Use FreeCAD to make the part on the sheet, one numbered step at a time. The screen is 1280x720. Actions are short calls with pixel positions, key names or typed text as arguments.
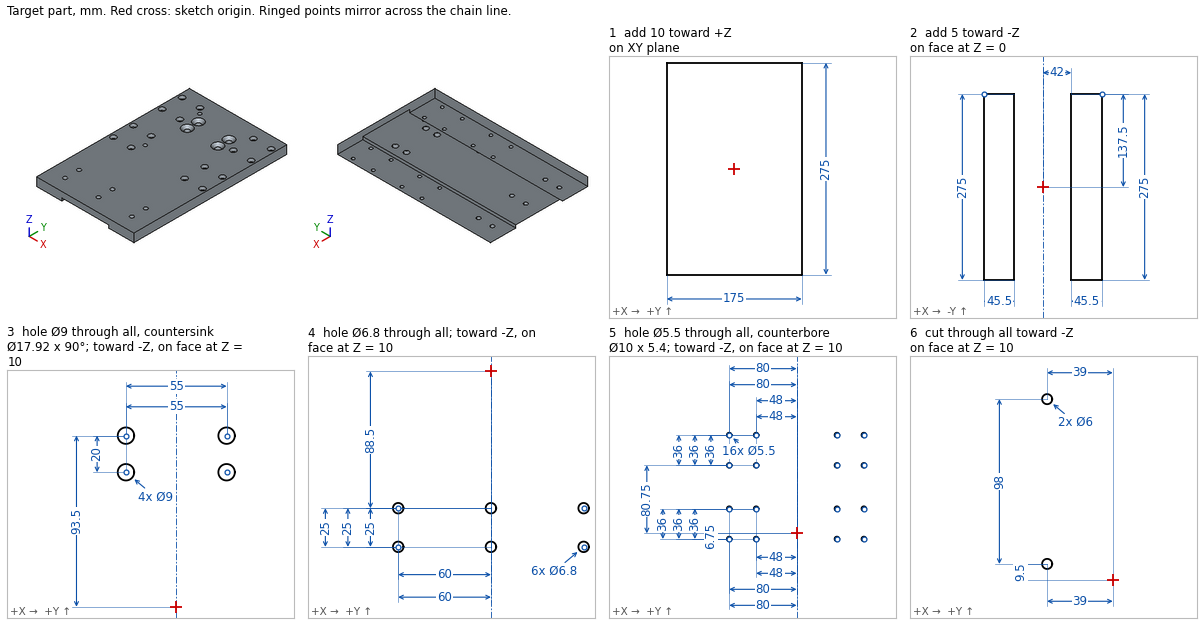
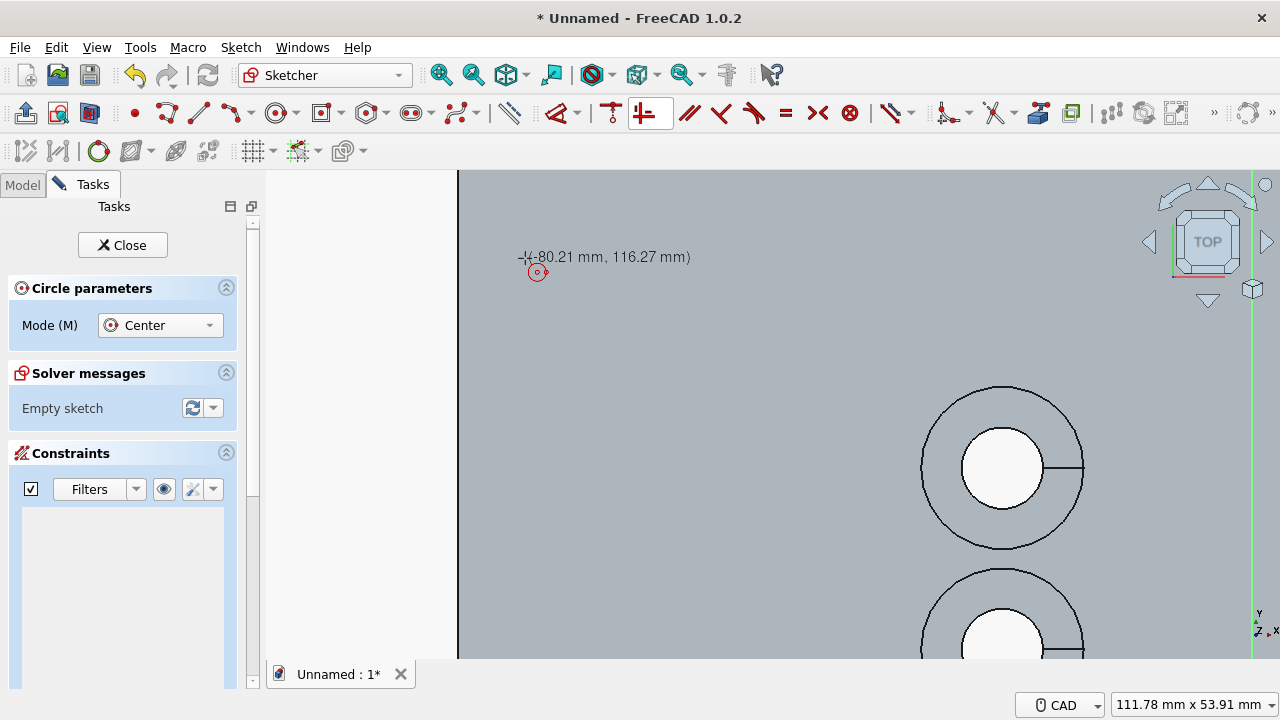
scroll(525, 283, down, 7)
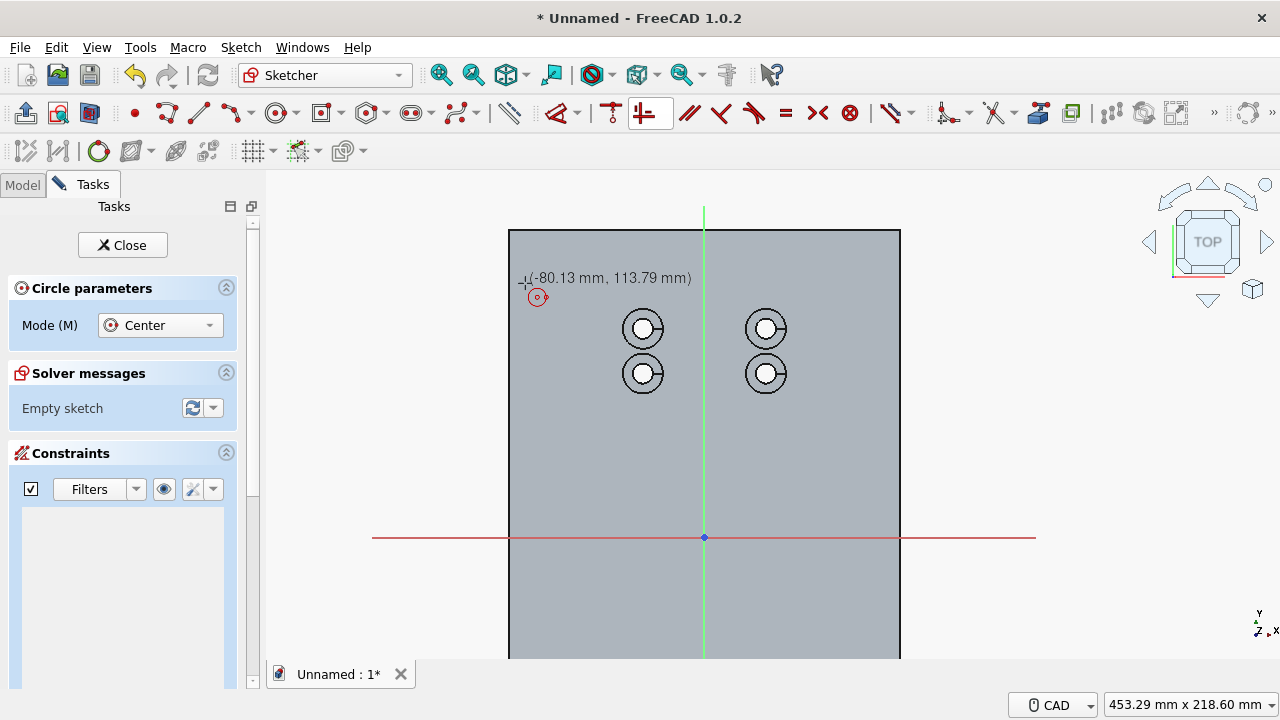
click(525, 277)
move(530, 272)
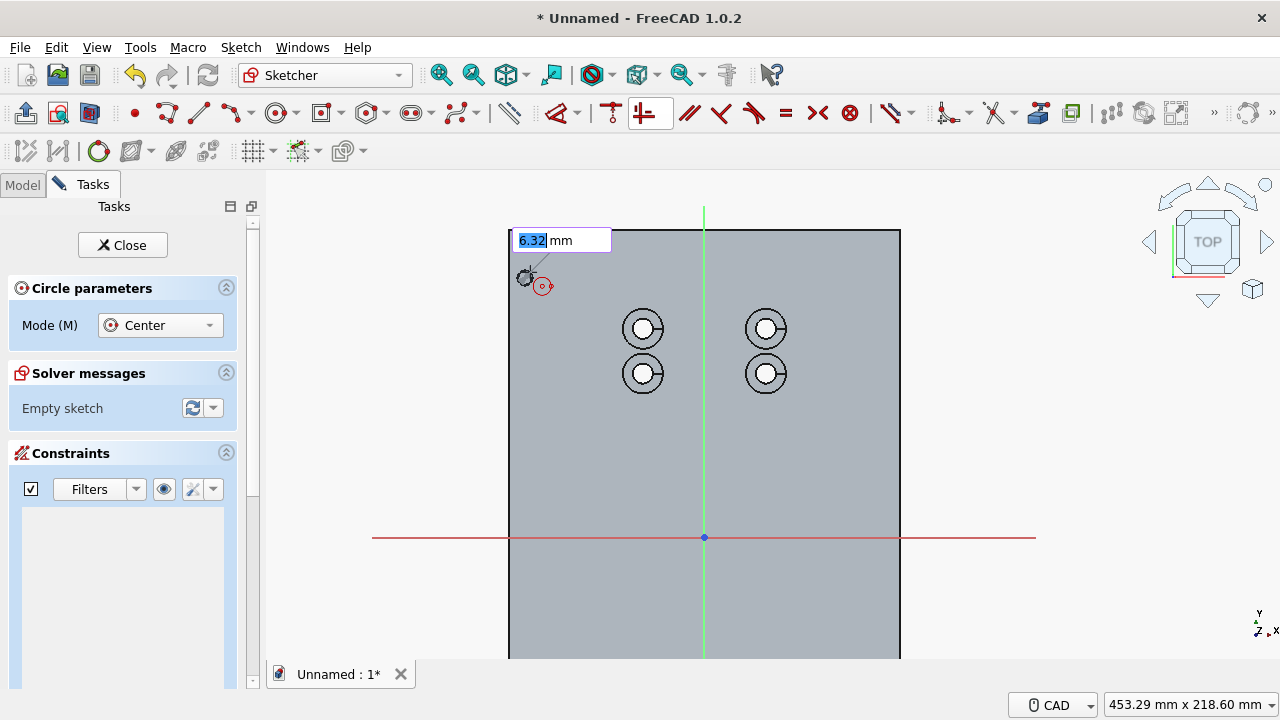
text(5.5)
key(Return)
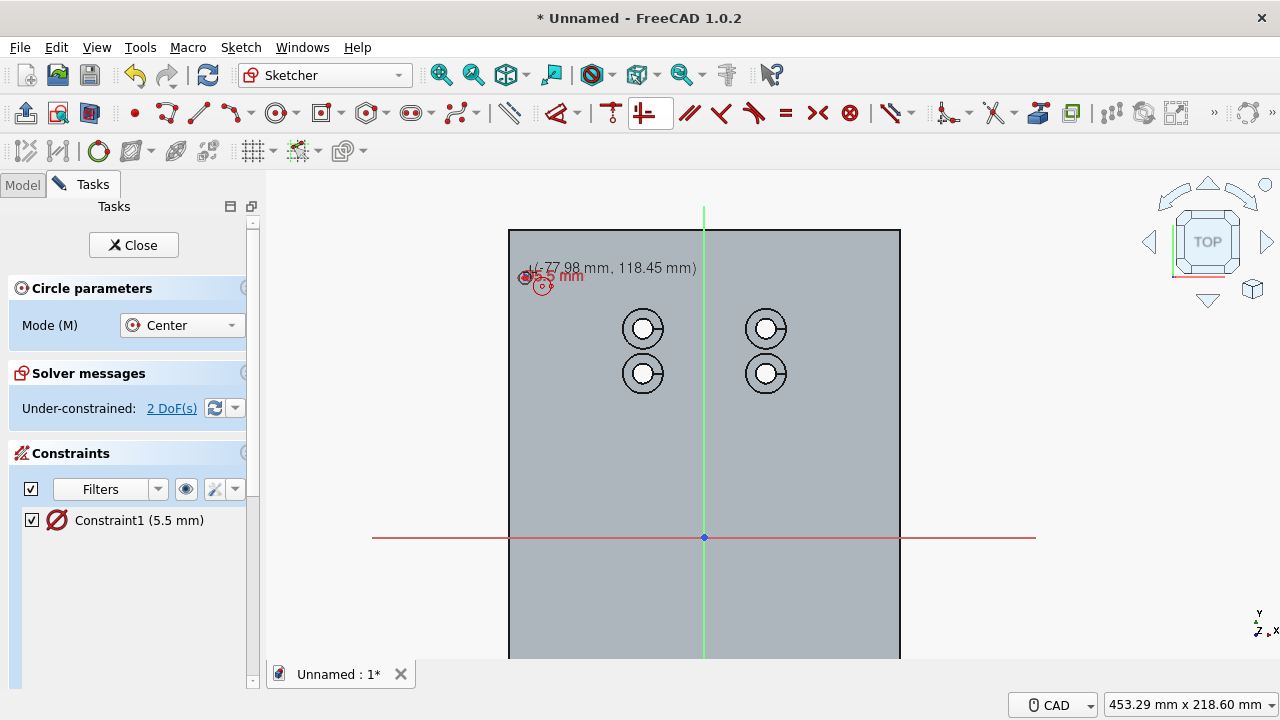
scroll(597, 277, up, 7)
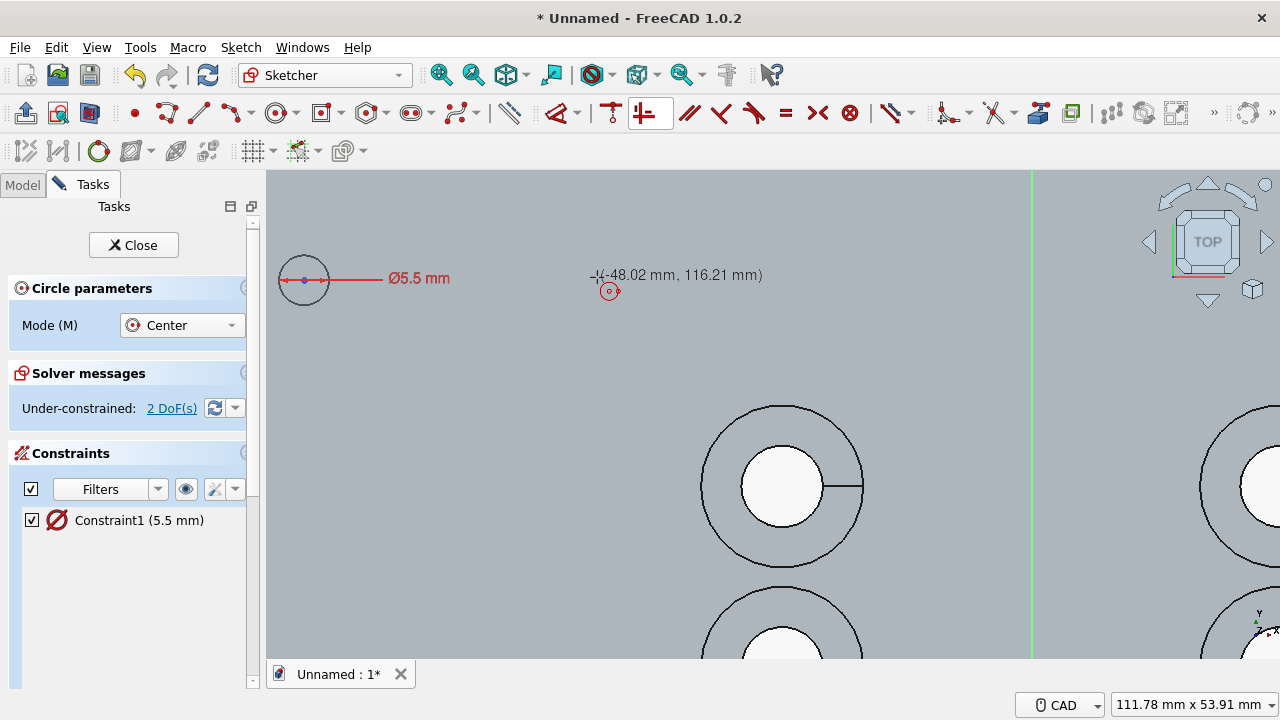
scroll(597, 277, down, 7)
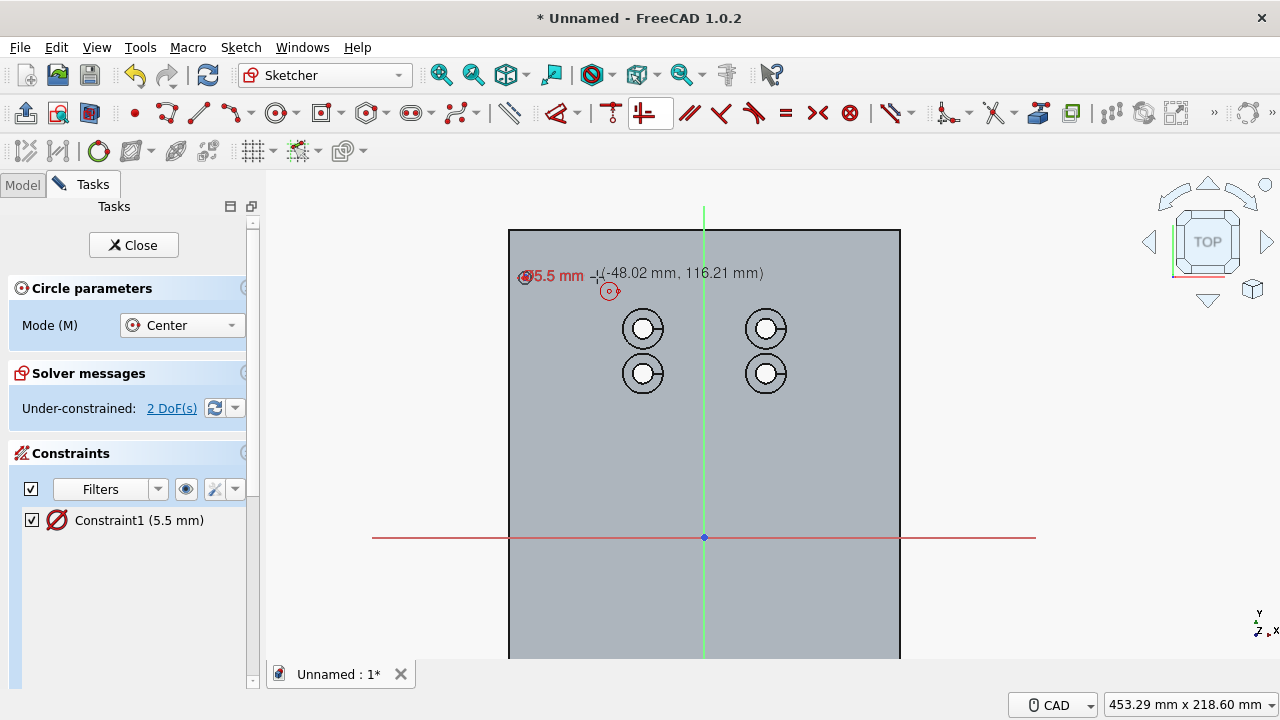
click(597, 277)
move(601, 272)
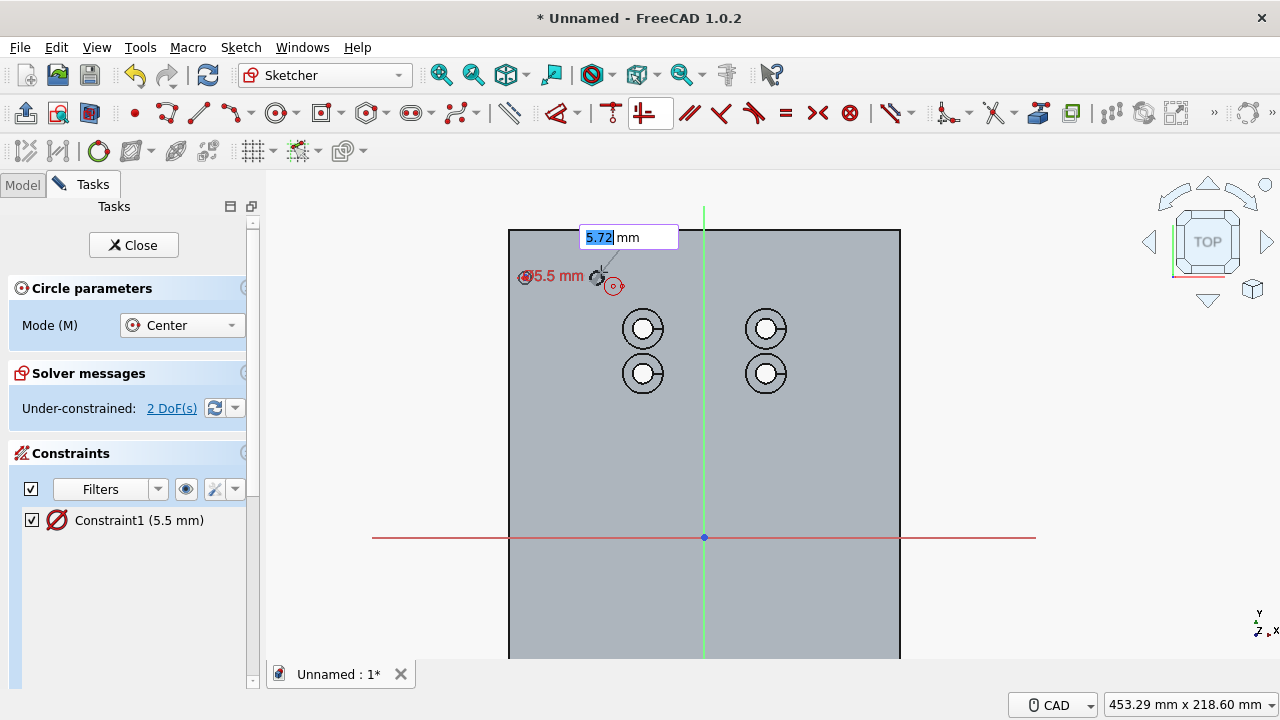
text(5.5)
key(Return)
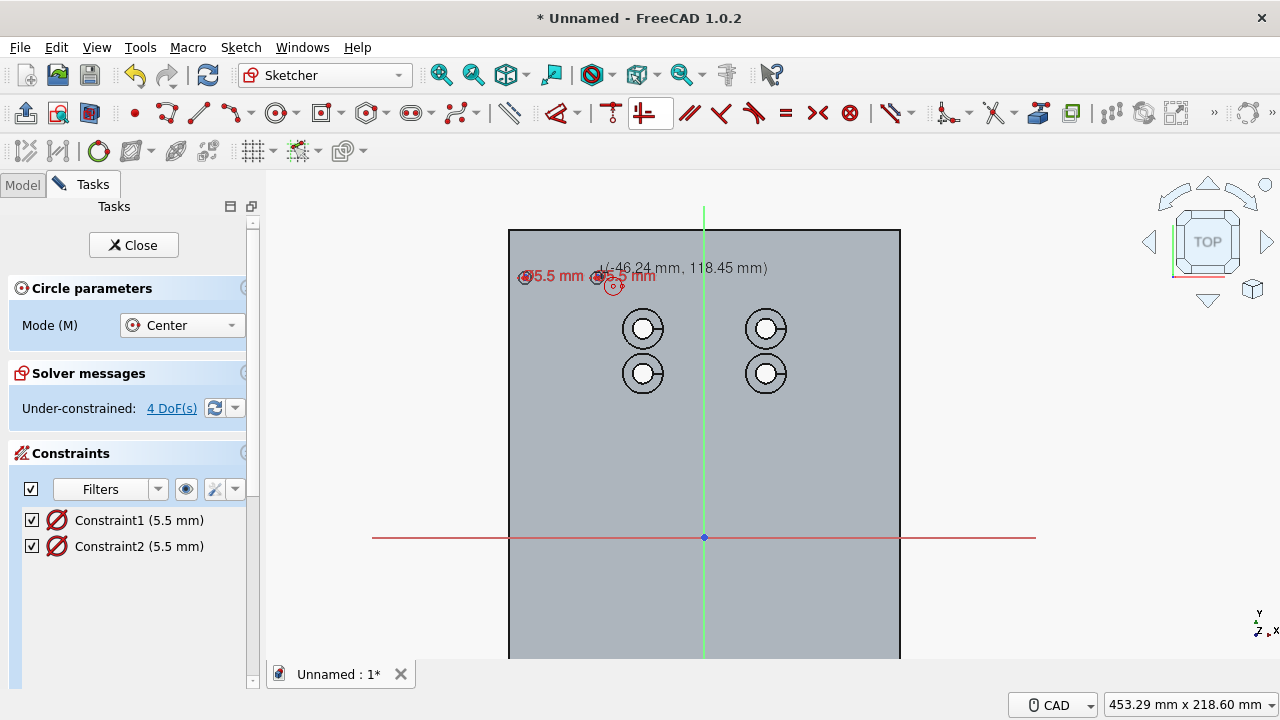
scroll(525, 357, up, 7)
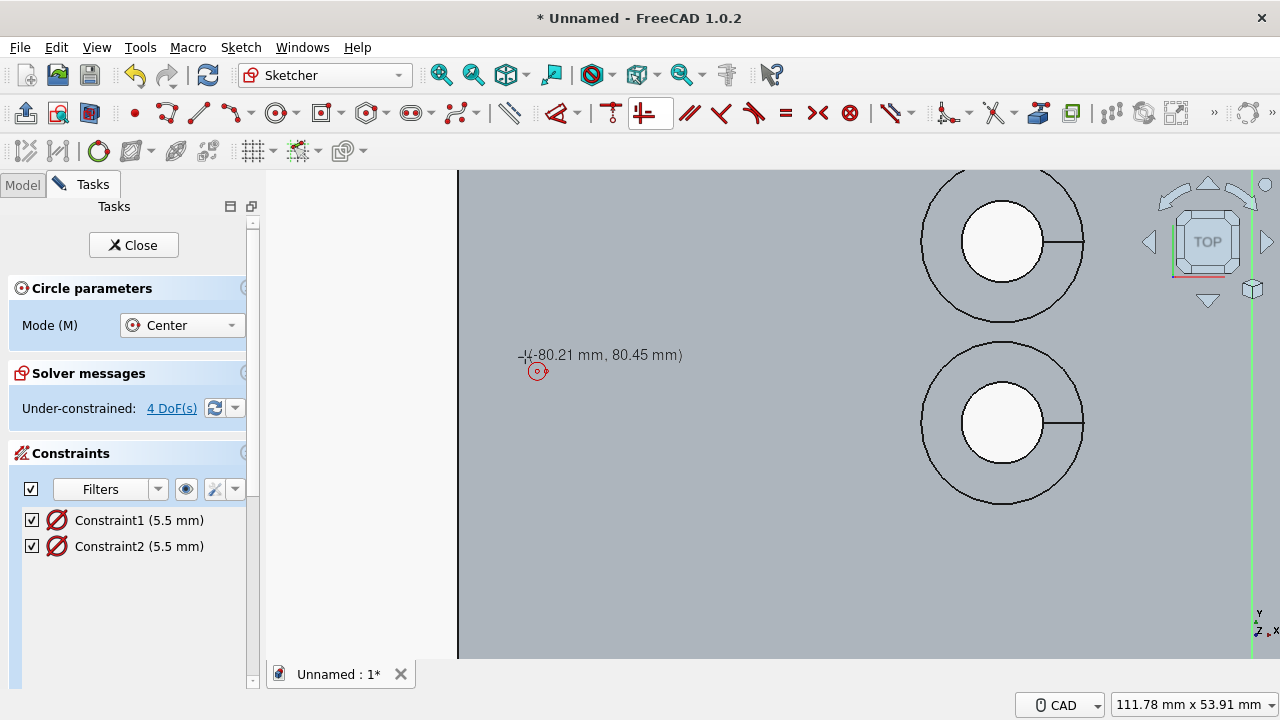
scroll(525, 357, down, 7)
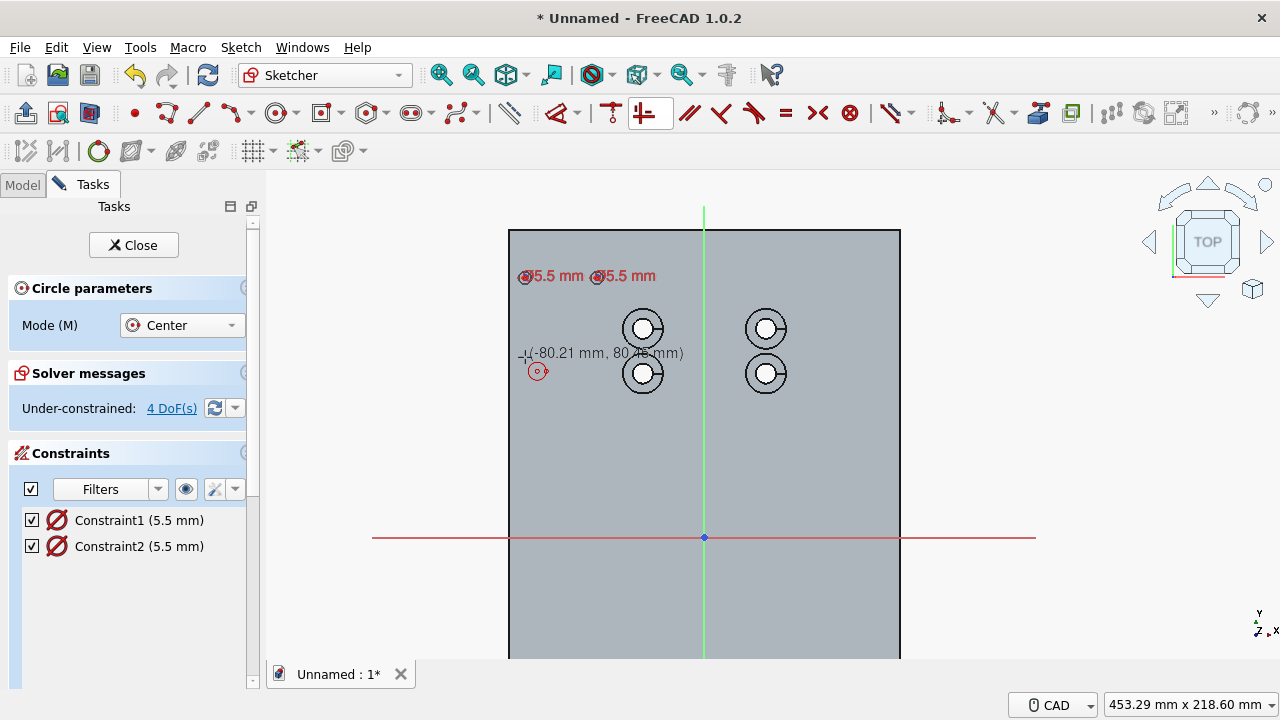
click(525, 357)
move(530, 353)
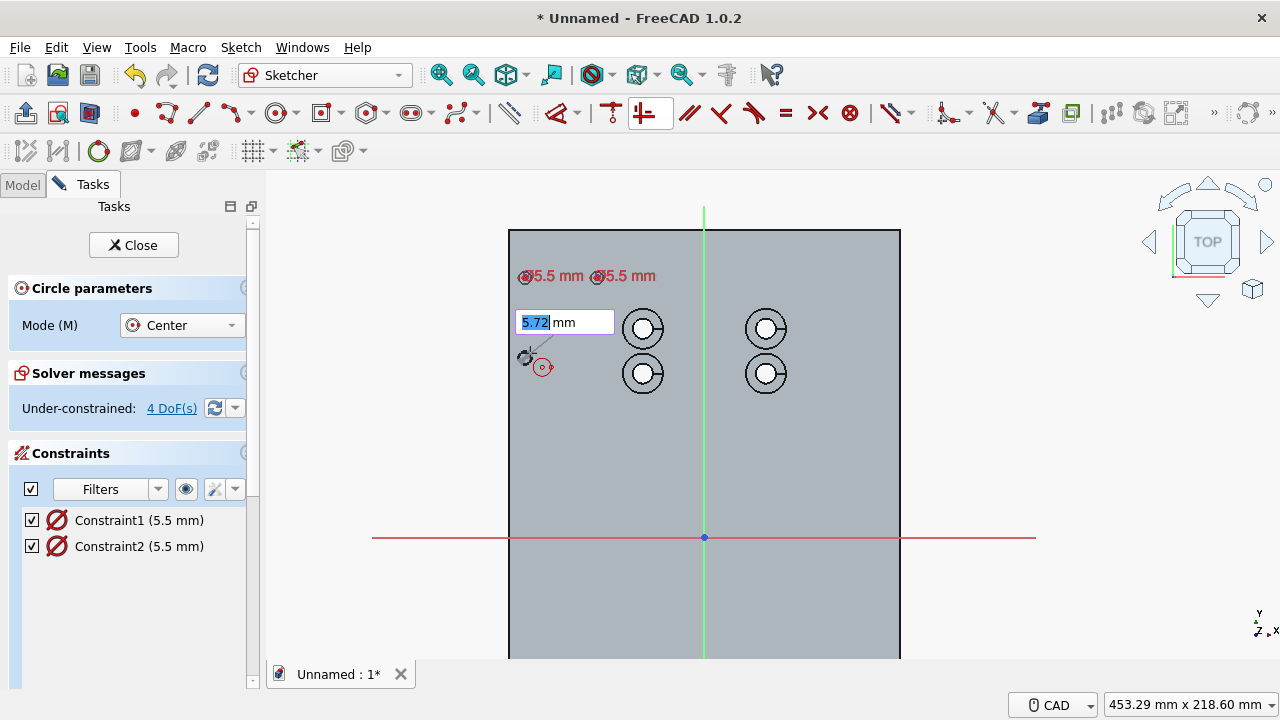
text(5.5)
key(Return)